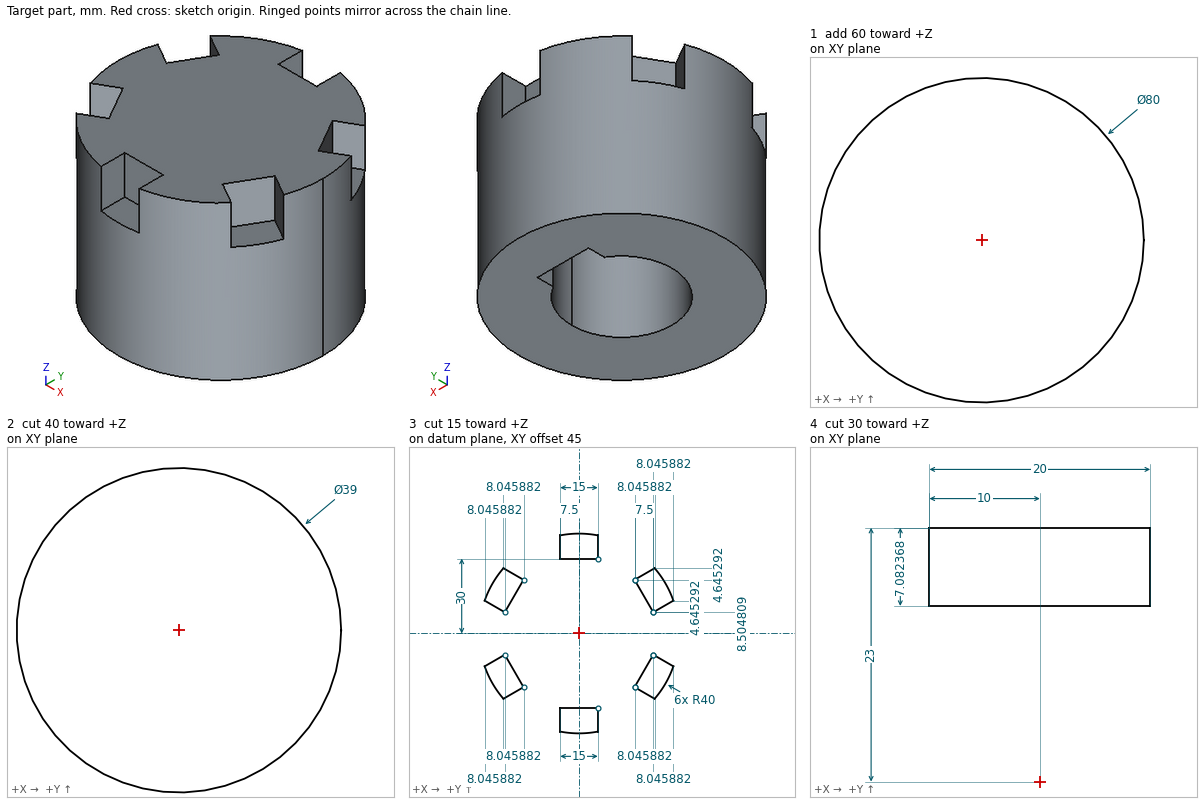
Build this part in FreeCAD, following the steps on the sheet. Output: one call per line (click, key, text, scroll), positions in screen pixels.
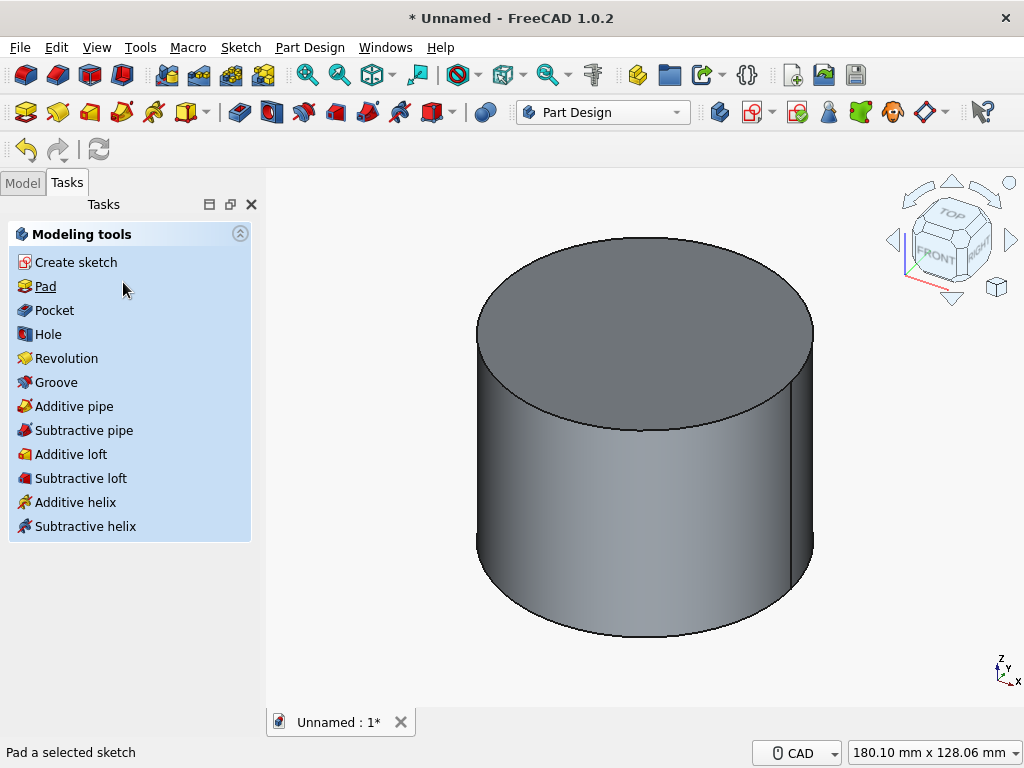
click(240, 112)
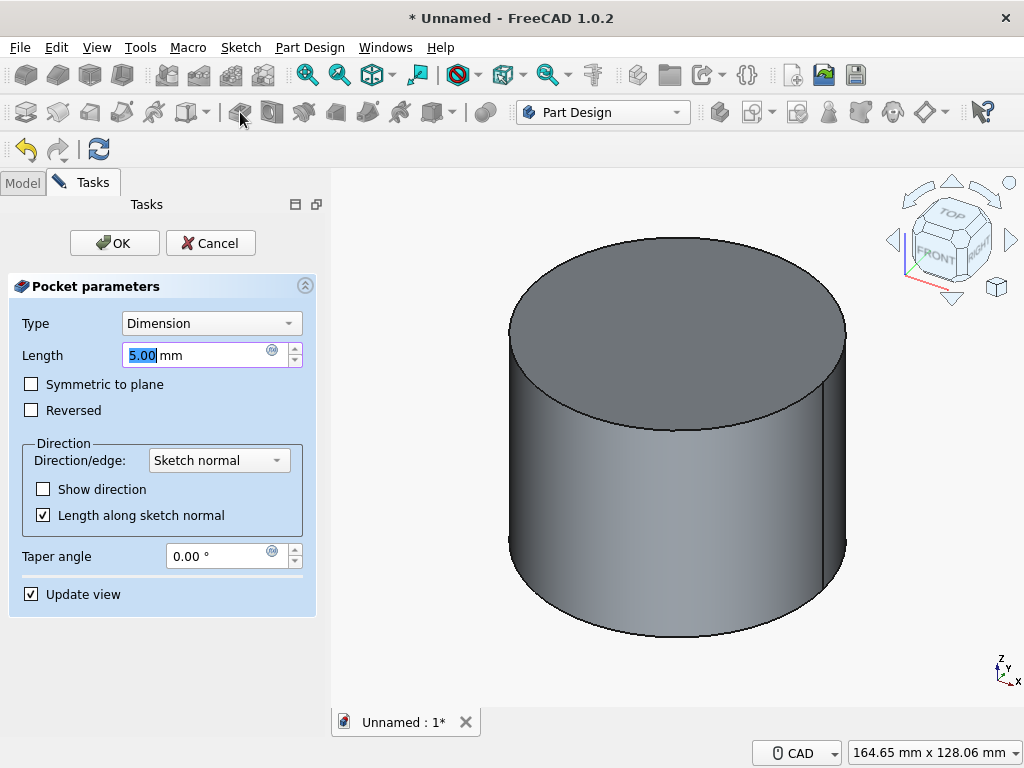
text(40)
key(Tab)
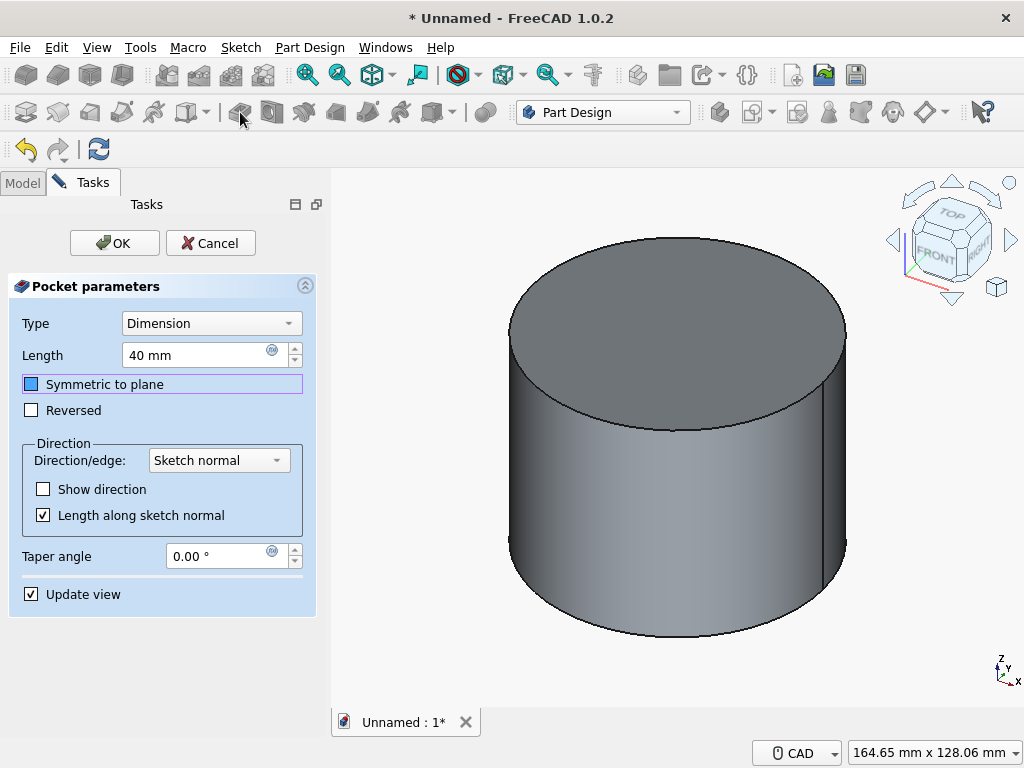
click(30, 410)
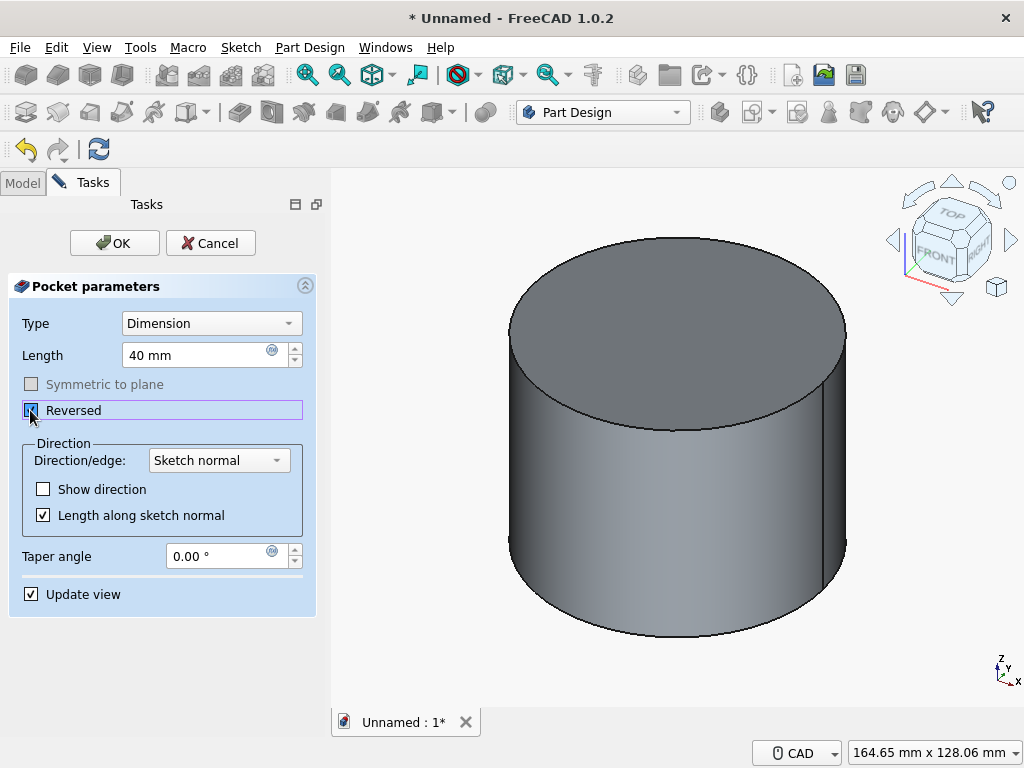
click(115, 243)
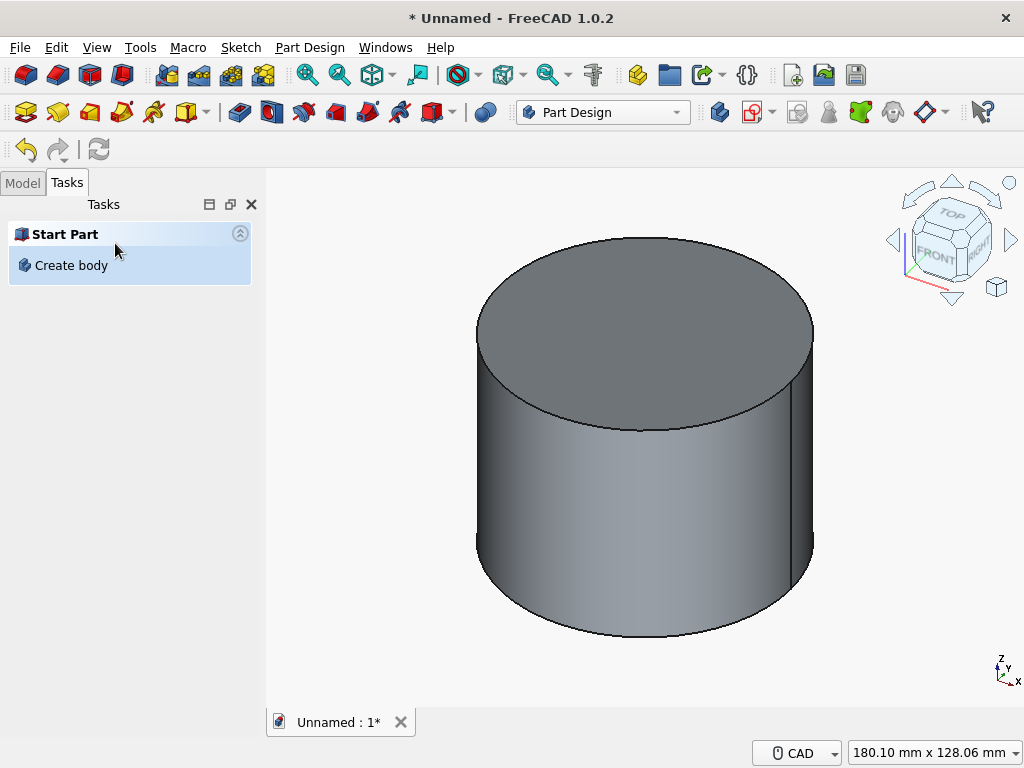
click(23, 182)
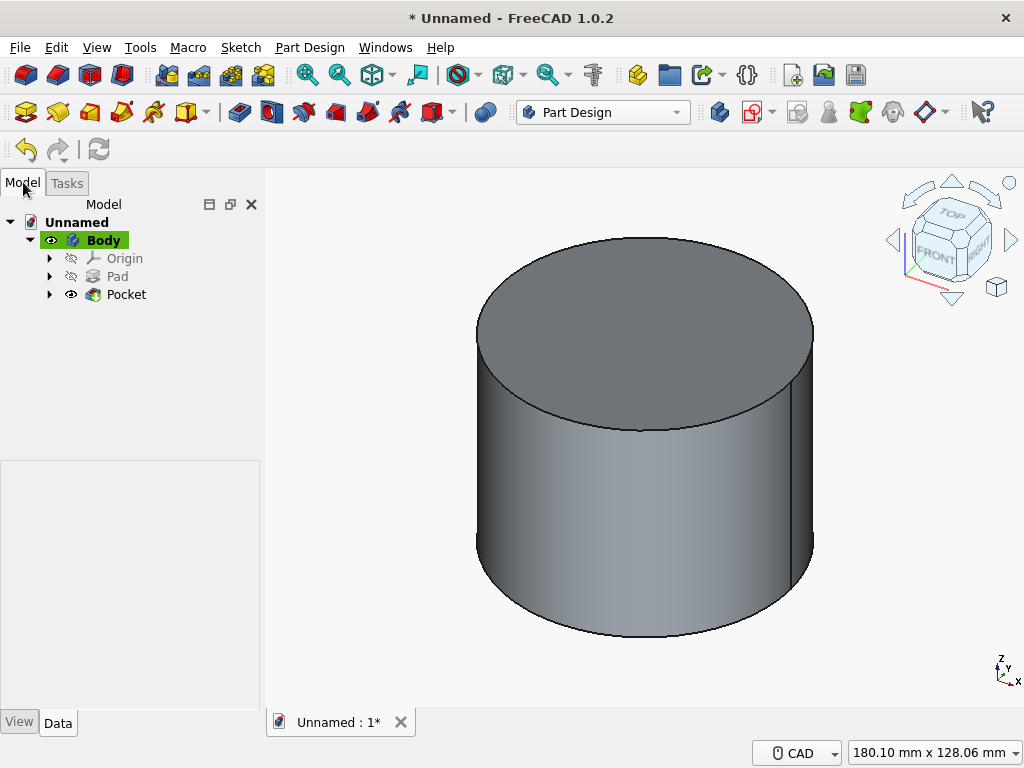
click(50, 258)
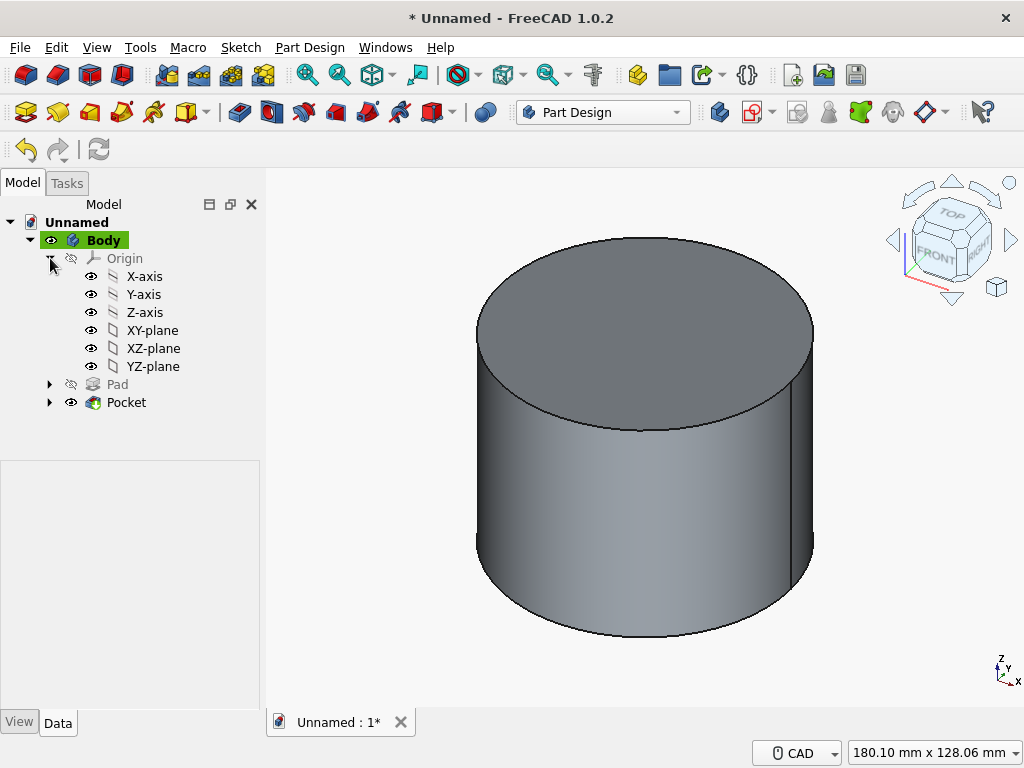
click(136, 330)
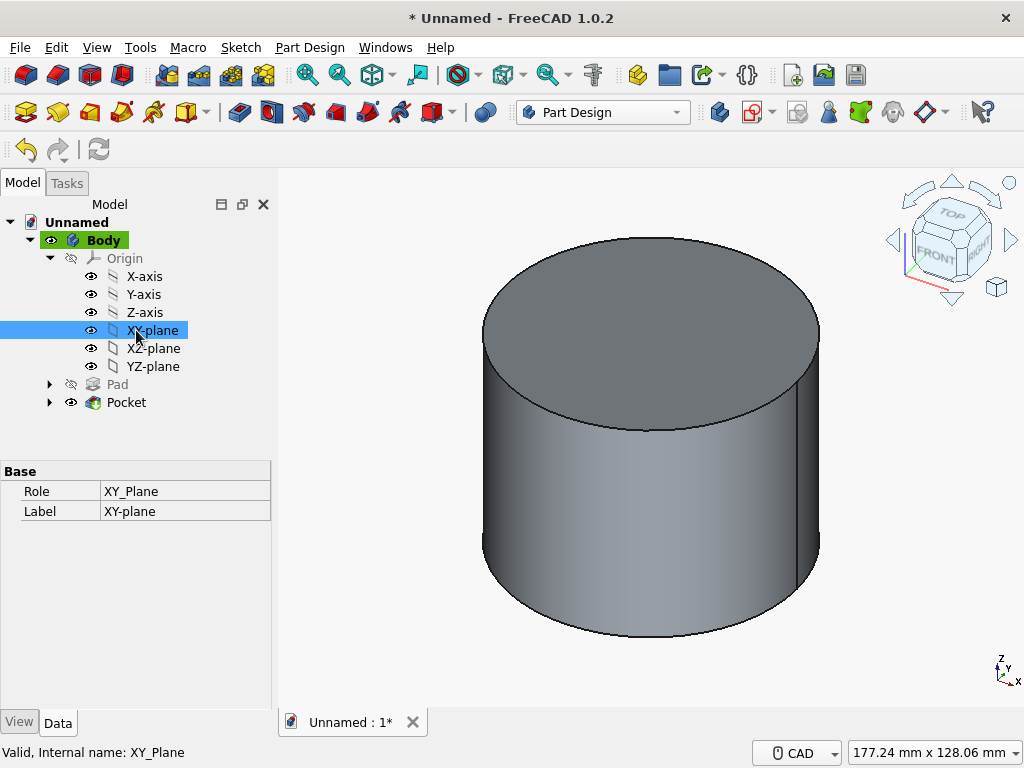
click(926, 112)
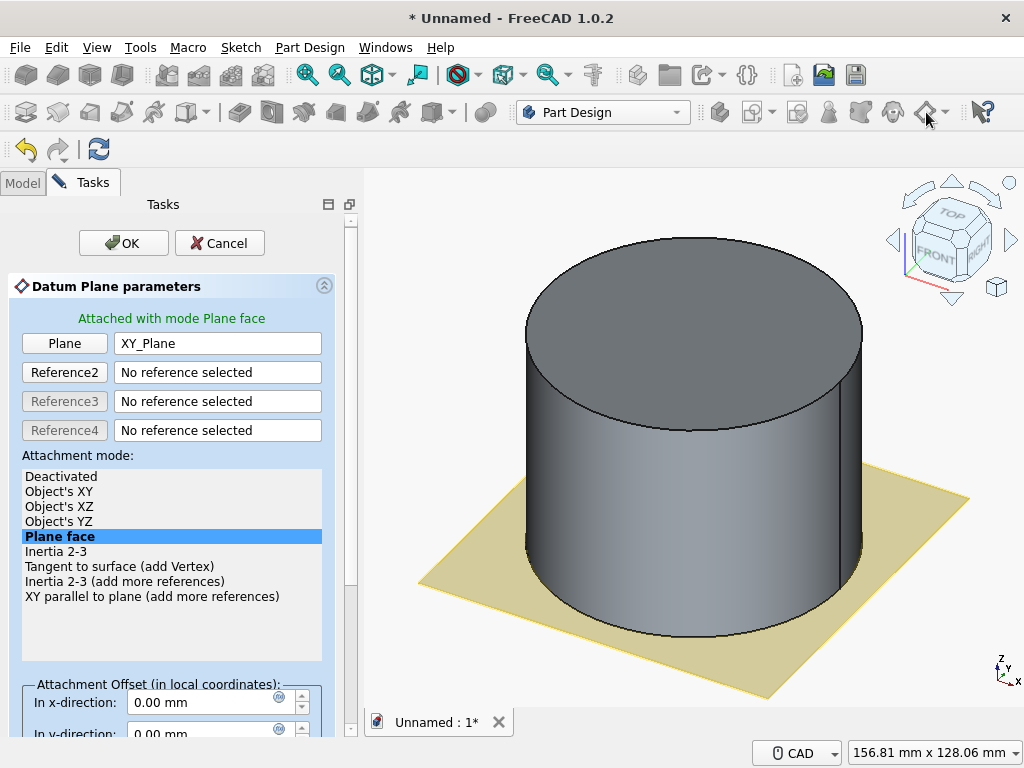
scroll(351, 475, down, 2)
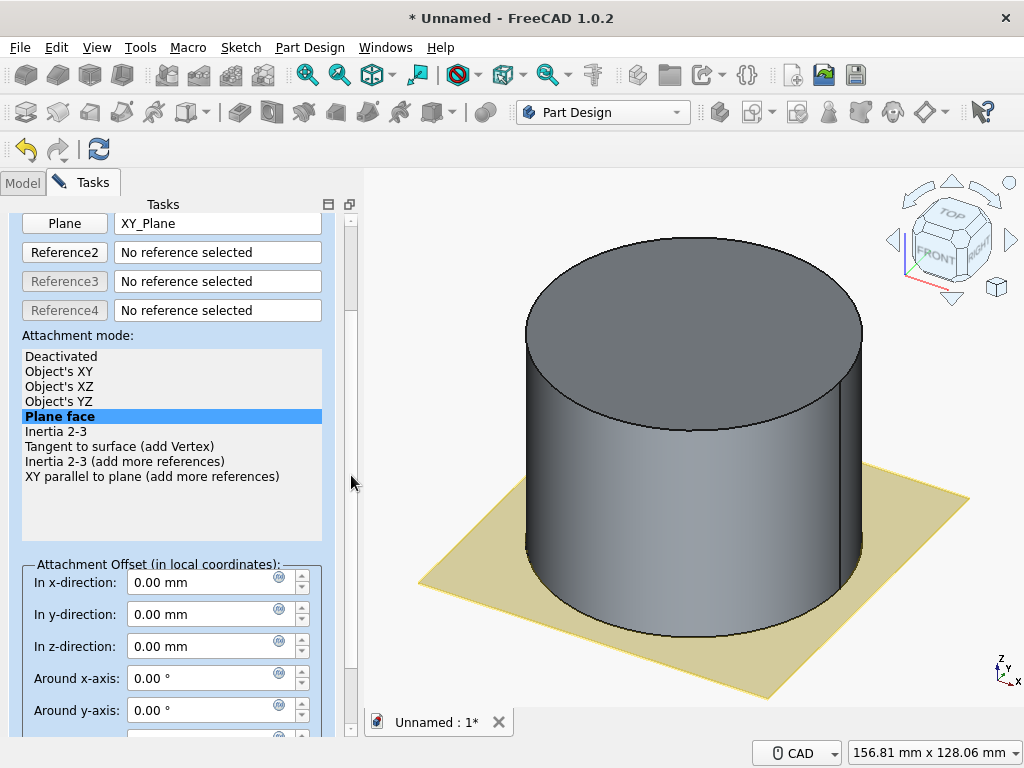
triple_click(210, 646)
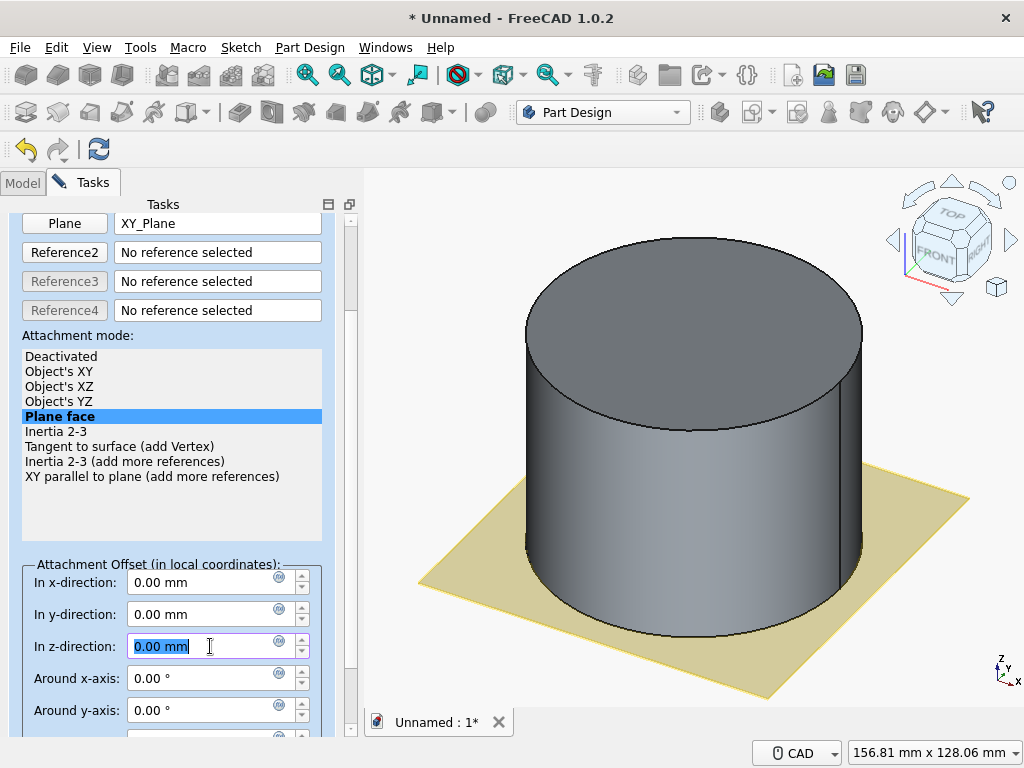
text(45)
key(Tab)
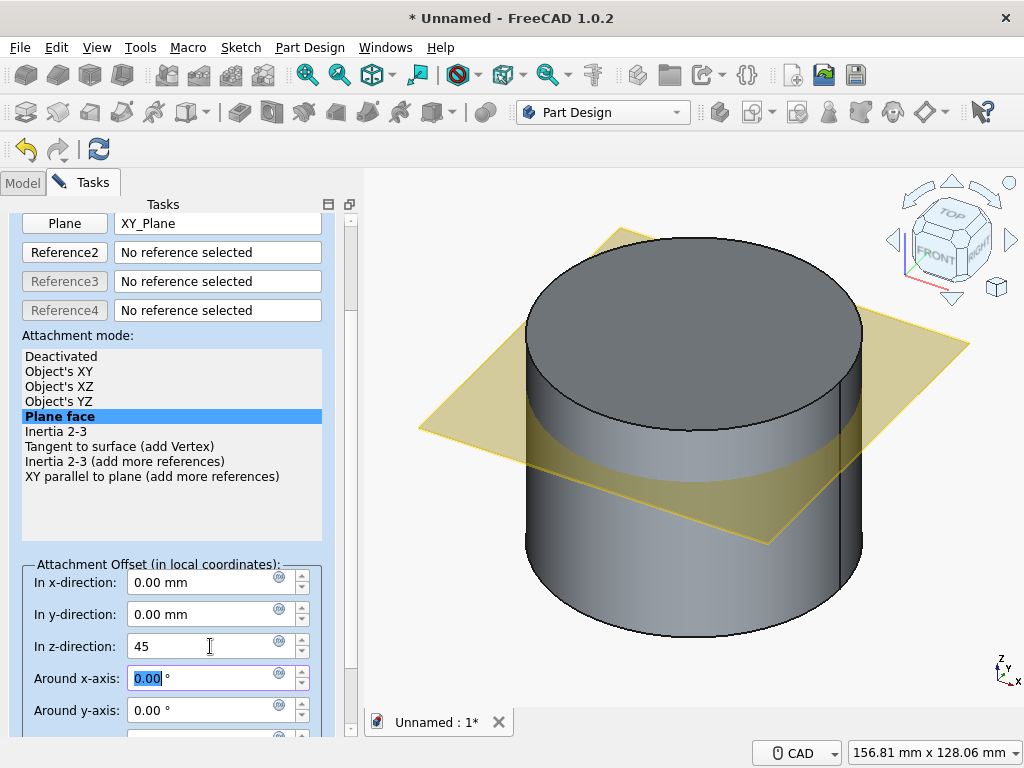
scroll(351, 475, up, 3)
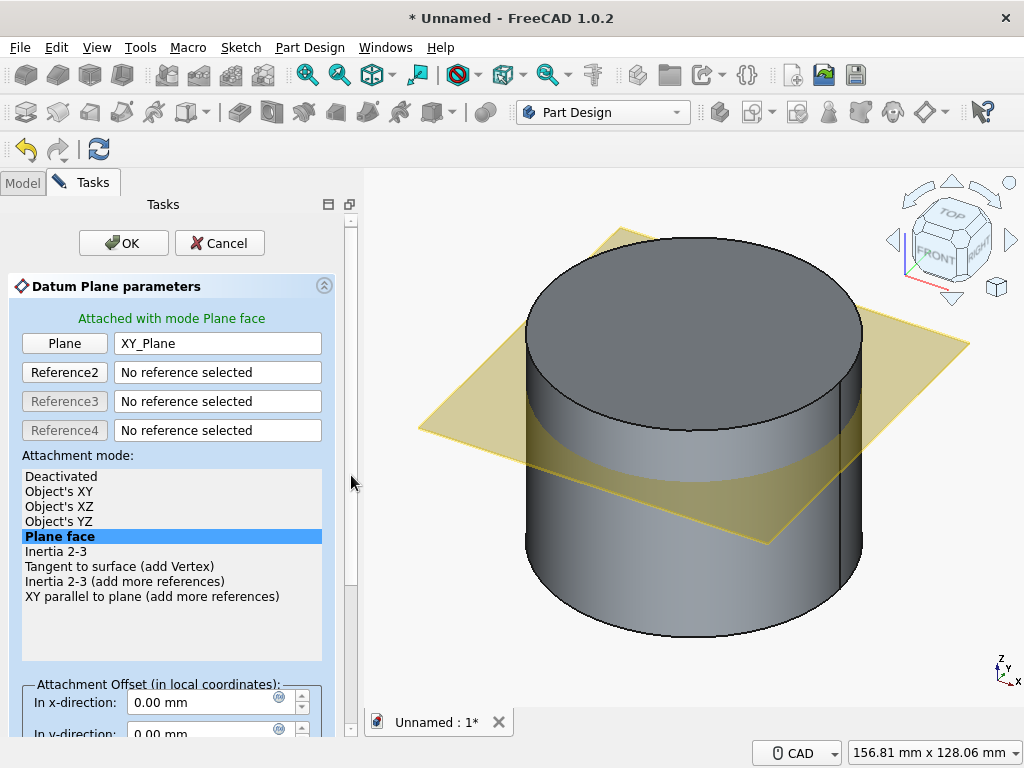
click(124, 243)